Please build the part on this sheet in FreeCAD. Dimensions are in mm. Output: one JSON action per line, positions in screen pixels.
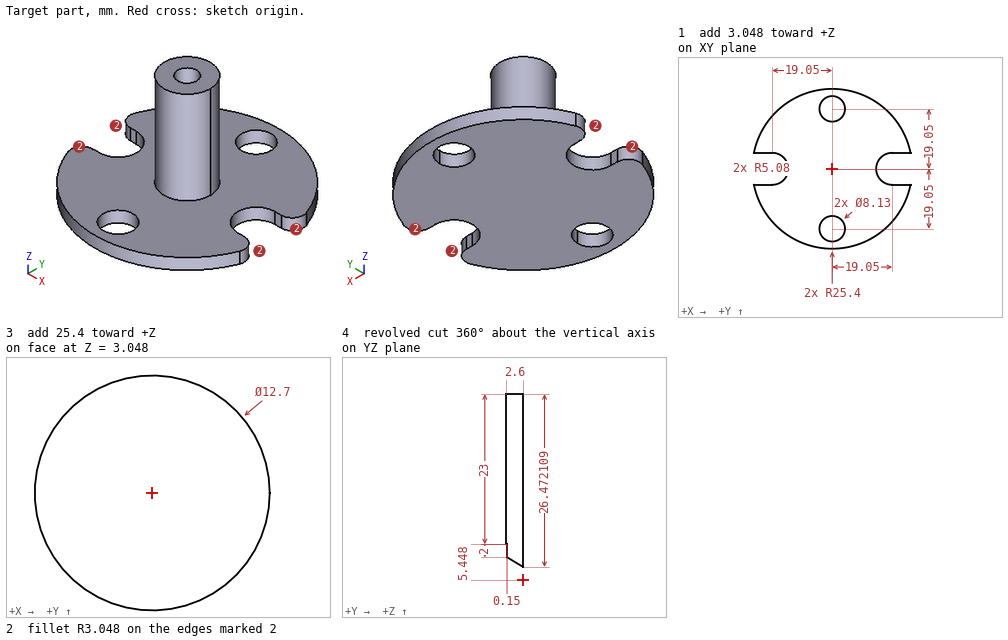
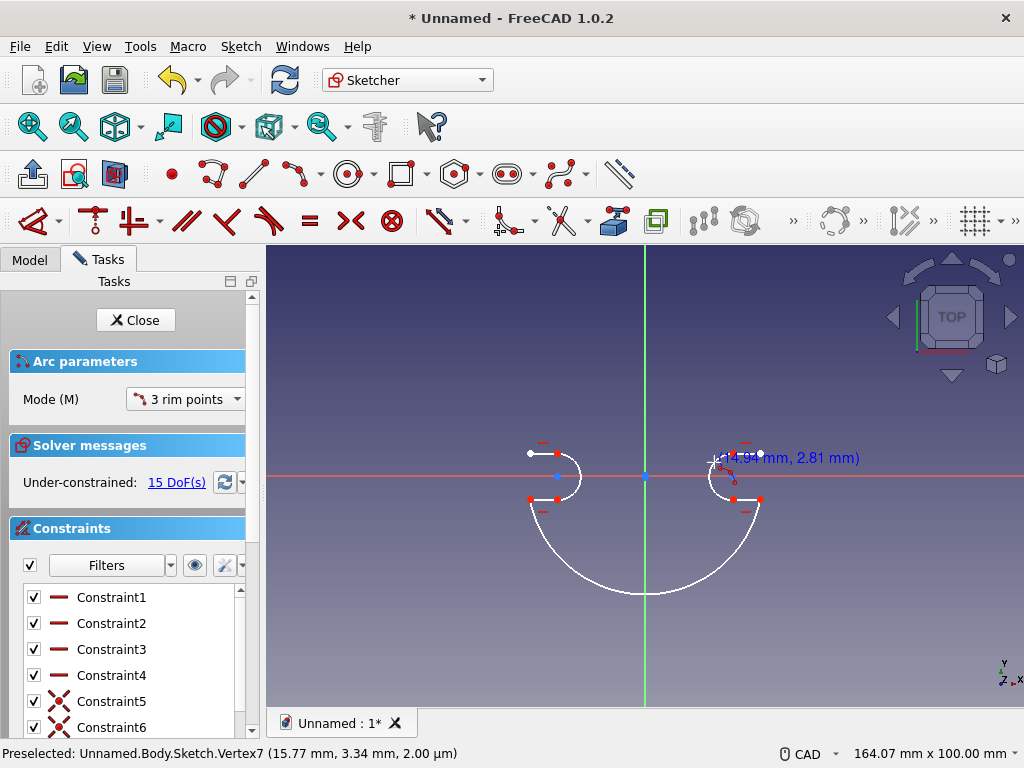
{"action": "left_click", "coordinate": [760, 454]}
{"action": "left_click", "coordinate": [530, 454]}
{"action": "left_click", "coordinate": [677, 363]}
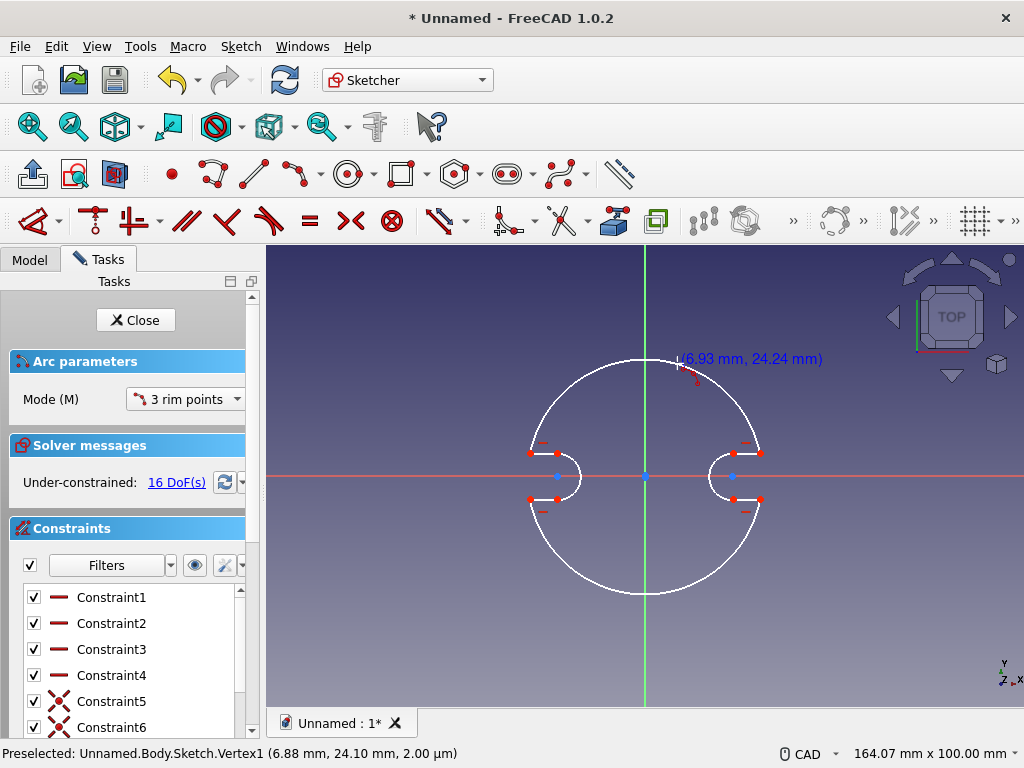
{"action": "left_click", "coordinate": [348, 174]}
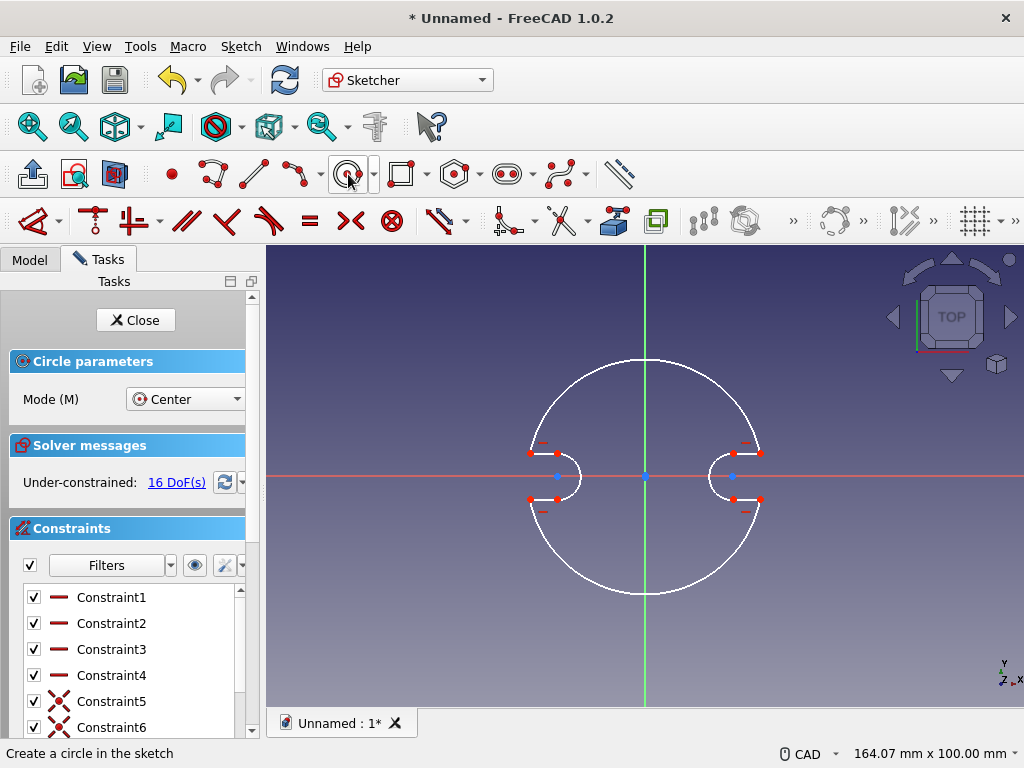
{"action": "left_click", "coordinate": [645, 564]}
{"action": "mouse_move", "coordinate": [663, 558]}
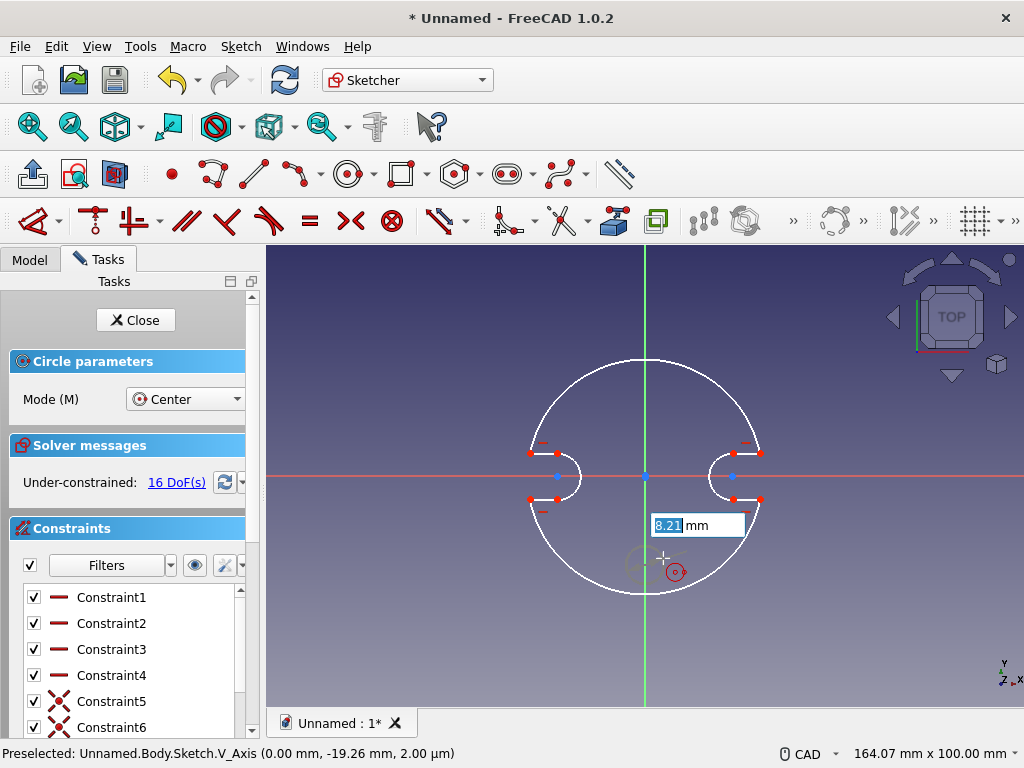
{"action": "type", "text": "8.13"}
{"action": "key", "text": "Return"}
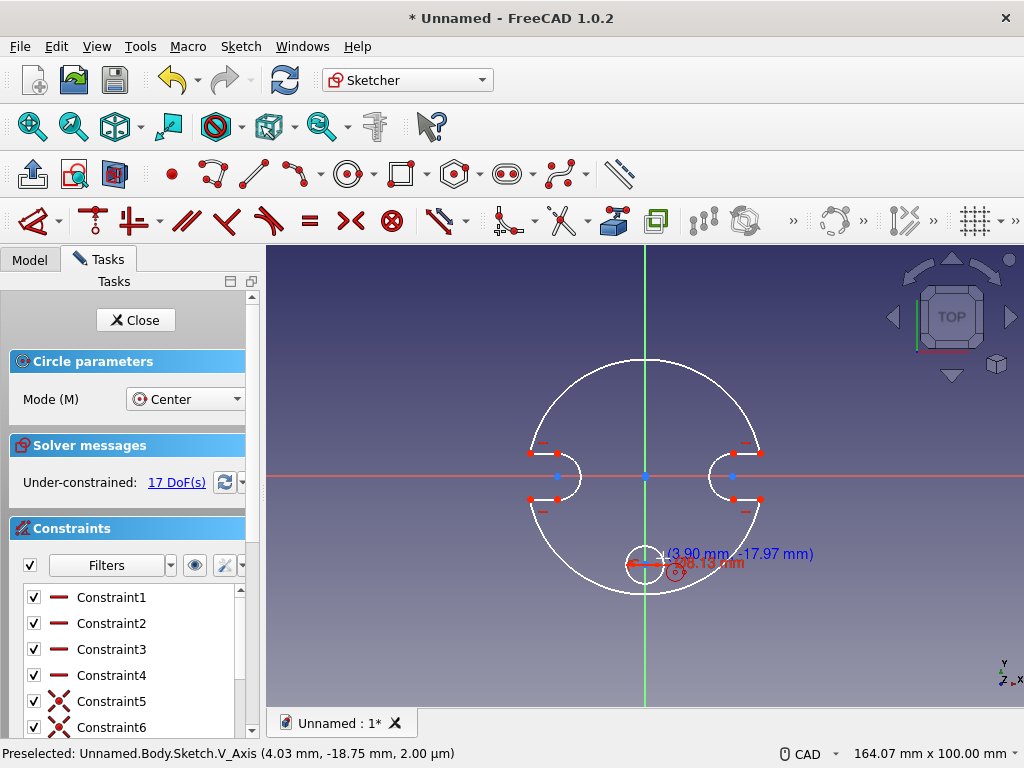
{"action": "left_click", "coordinate": [645, 388]}
{"action": "mouse_move", "coordinate": [663, 382]}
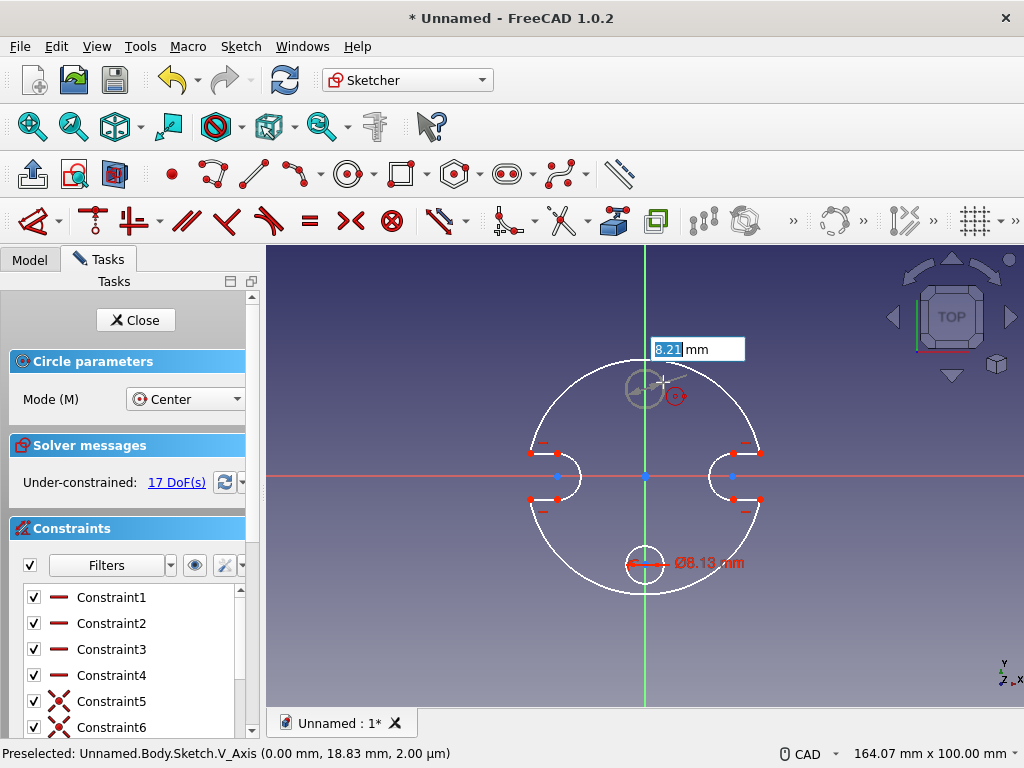
{"action": "type", "text": "8.13"}
{"action": "key", "text": "Return"}
{"action": "key", "text": "Escape"}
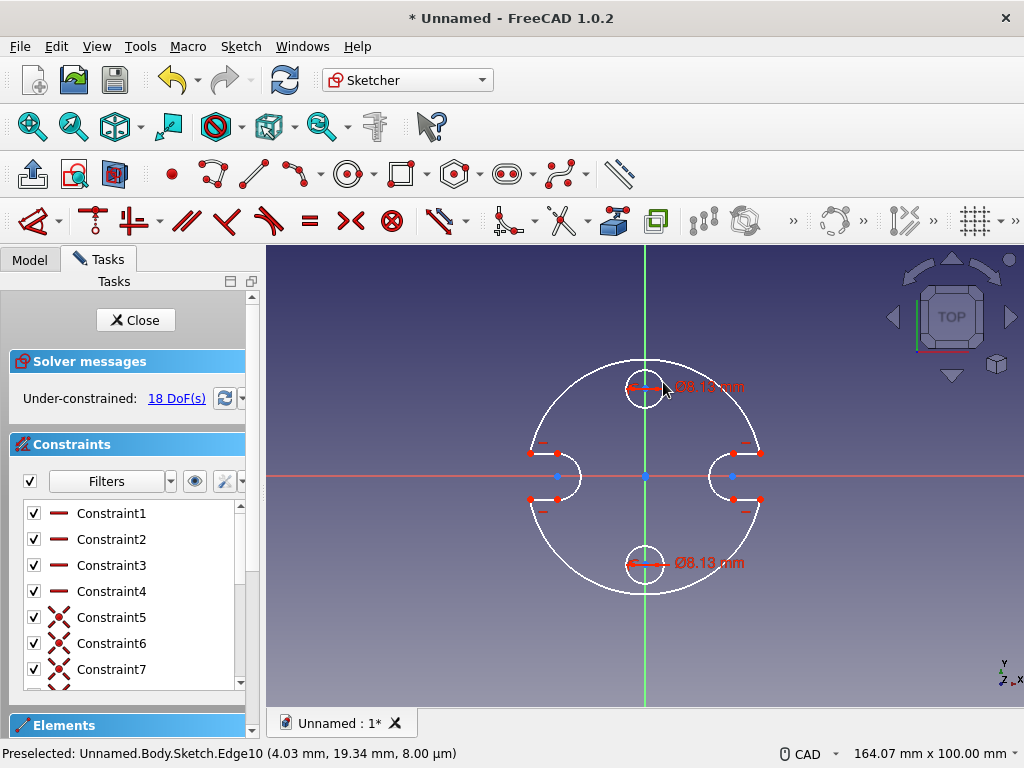
{"action": "scroll", "coordinate": [541, 454], "scroll_direction": "up", "scroll_amount": 2}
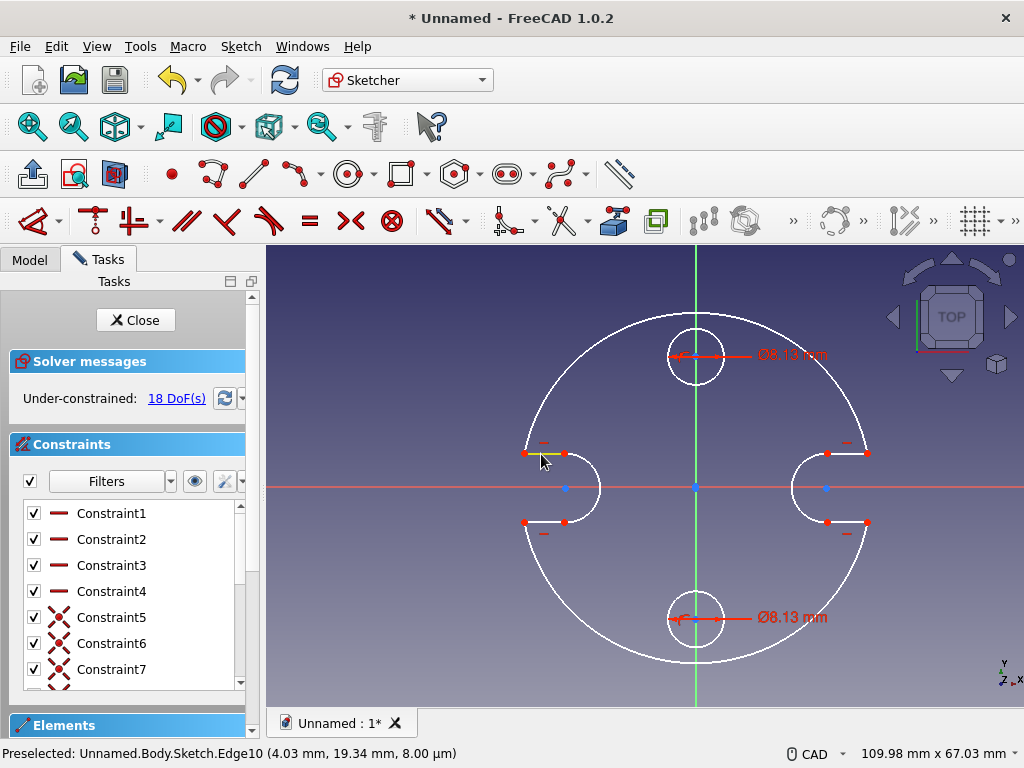
{"action": "left_click", "coordinate": [541, 454]}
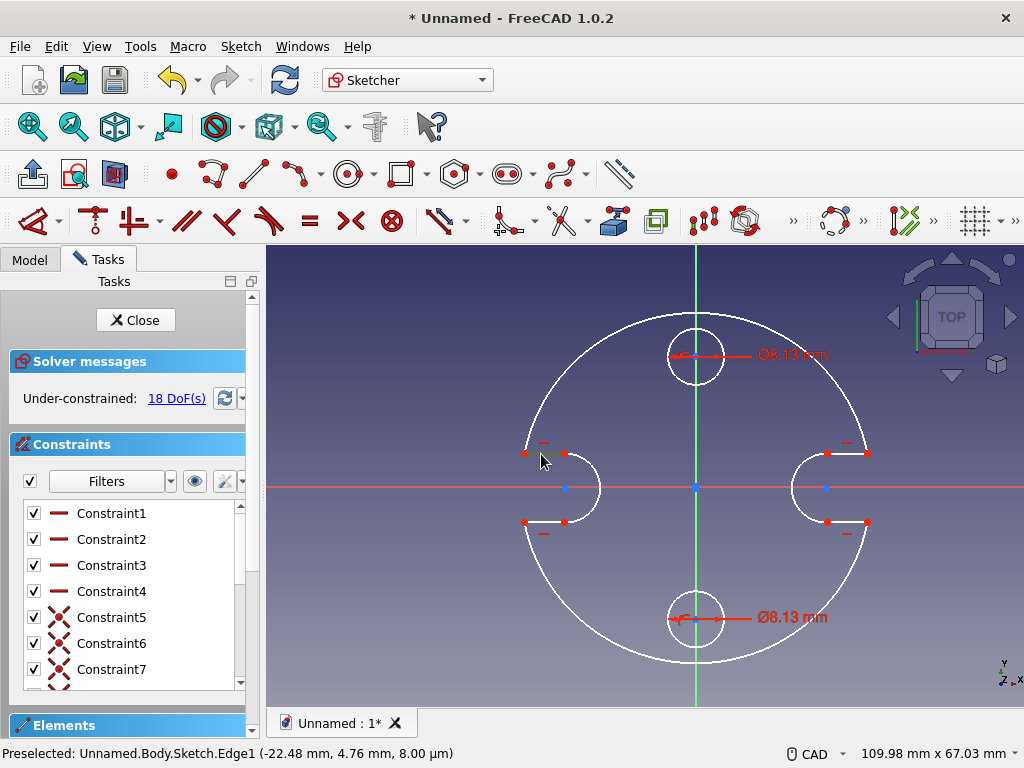
{"action": "left_click", "coordinate": [593, 509]}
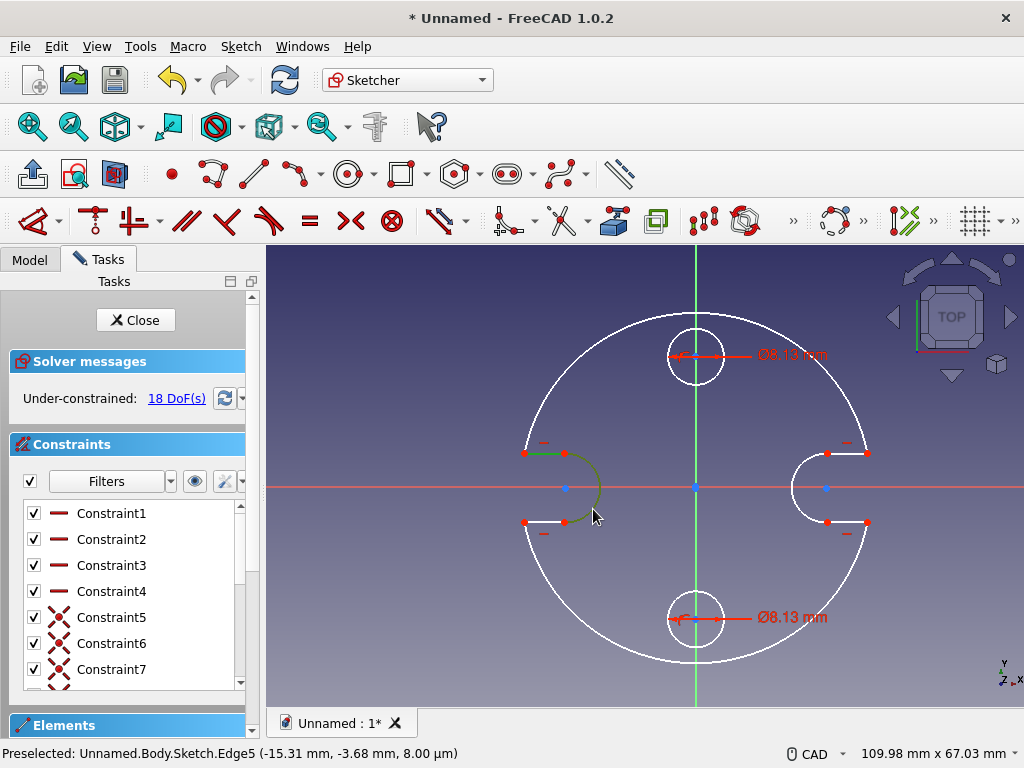
{"action": "left_click", "coordinate": [269, 222]}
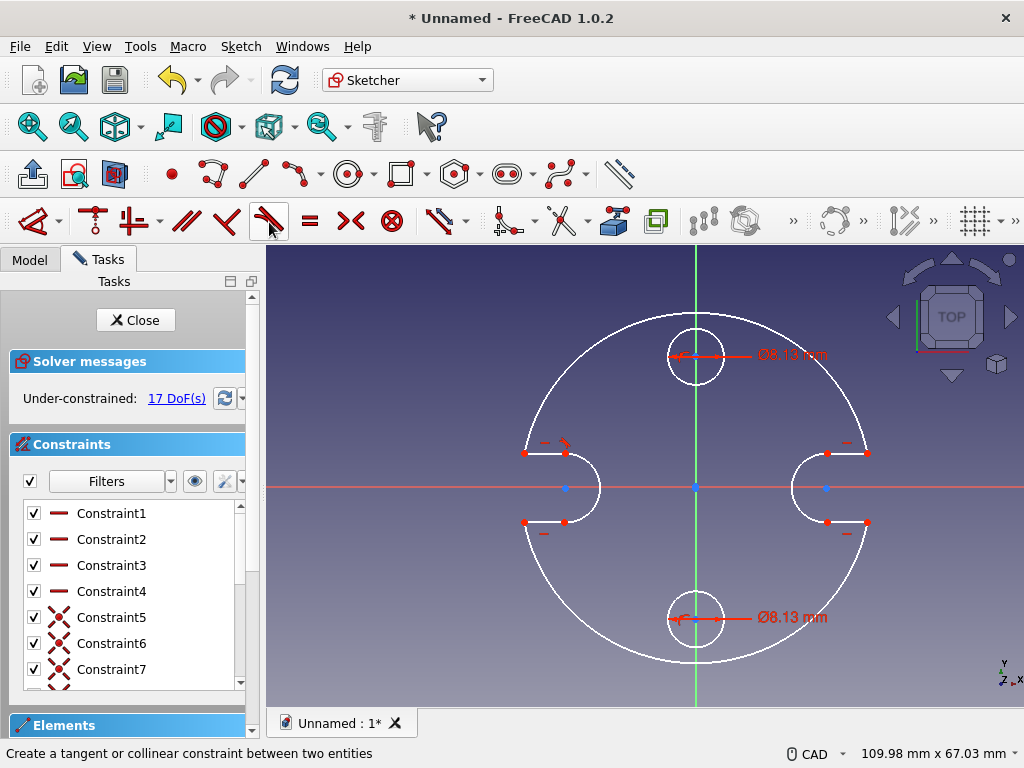
{"action": "left_click", "coordinate": [553, 522]}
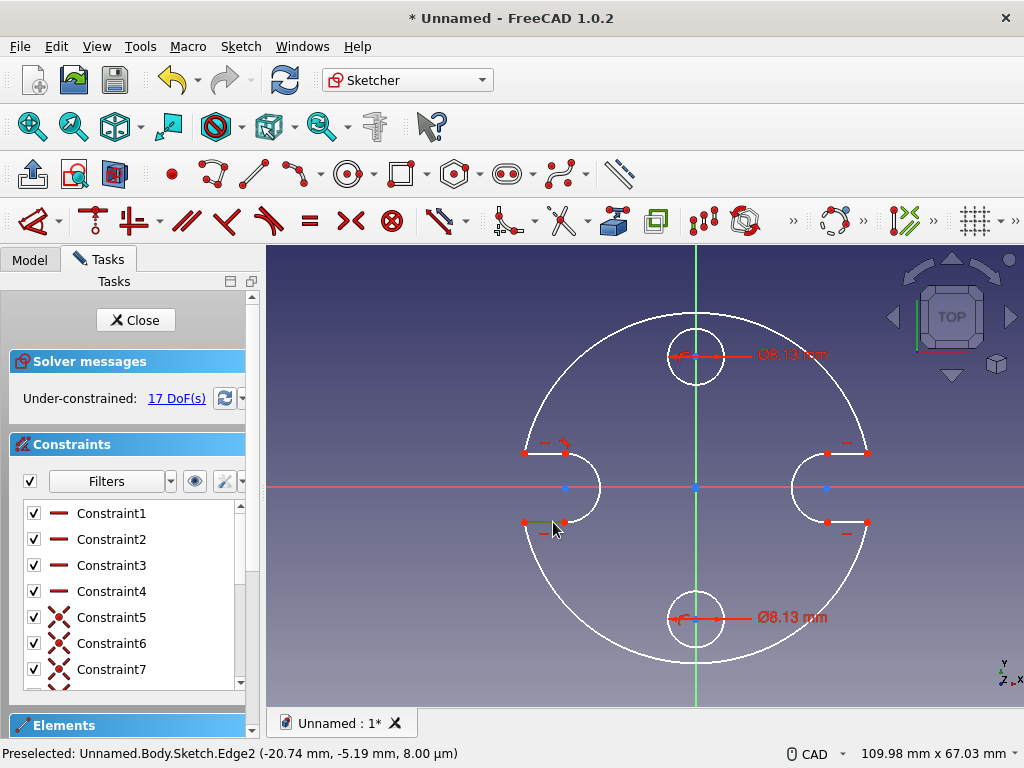
{"action": "left_click", "coordinate": [593, 509]}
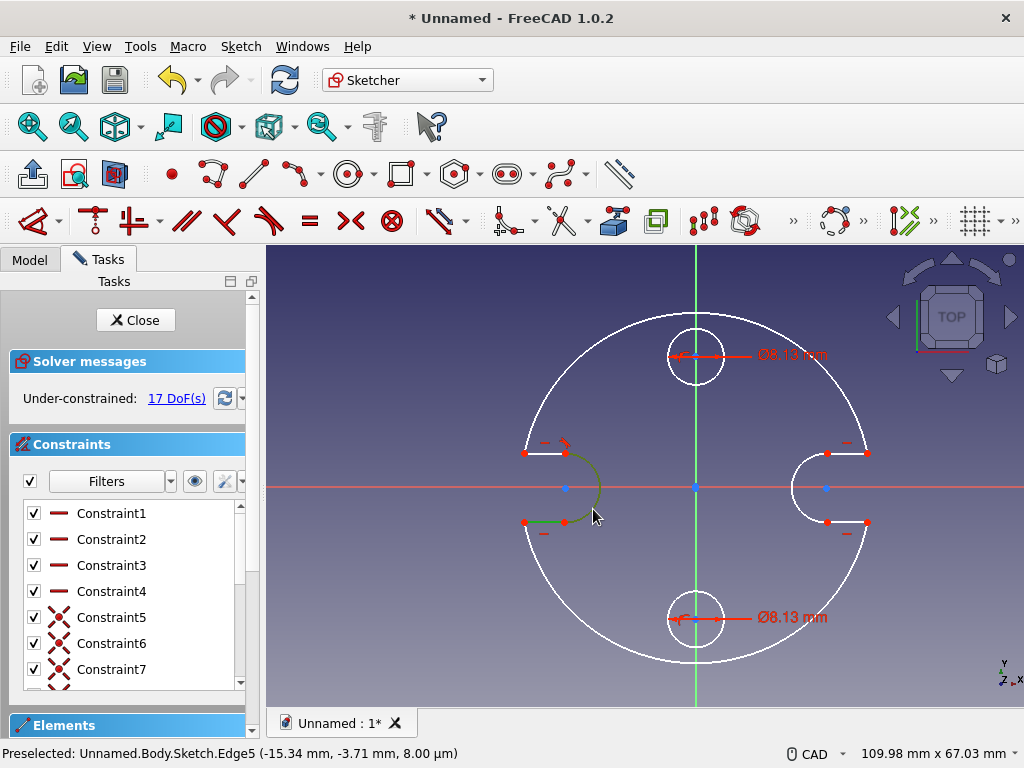
{"action": "left_click", "coordinate": [269, 222]}